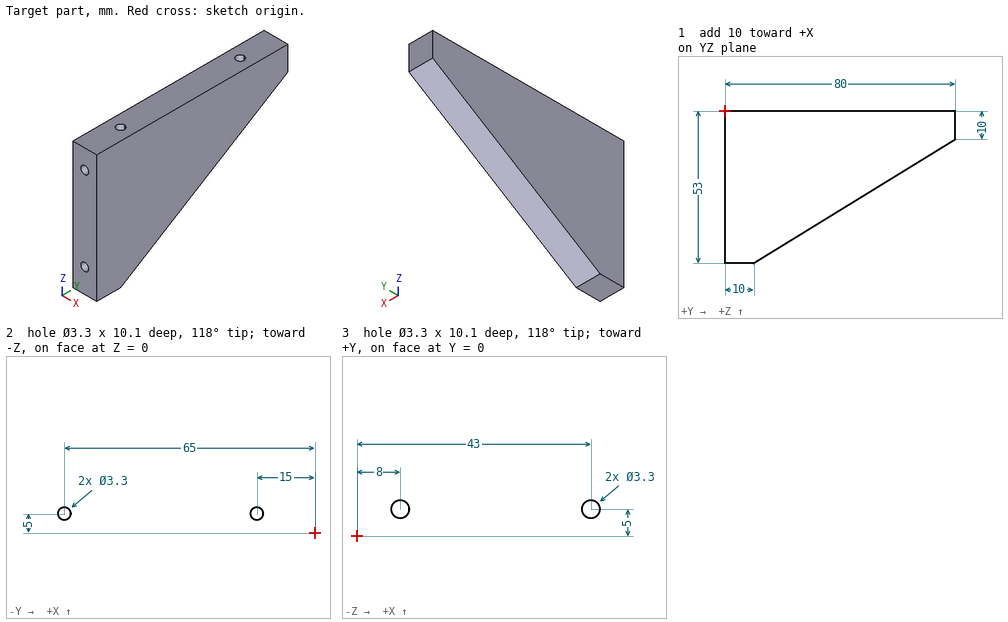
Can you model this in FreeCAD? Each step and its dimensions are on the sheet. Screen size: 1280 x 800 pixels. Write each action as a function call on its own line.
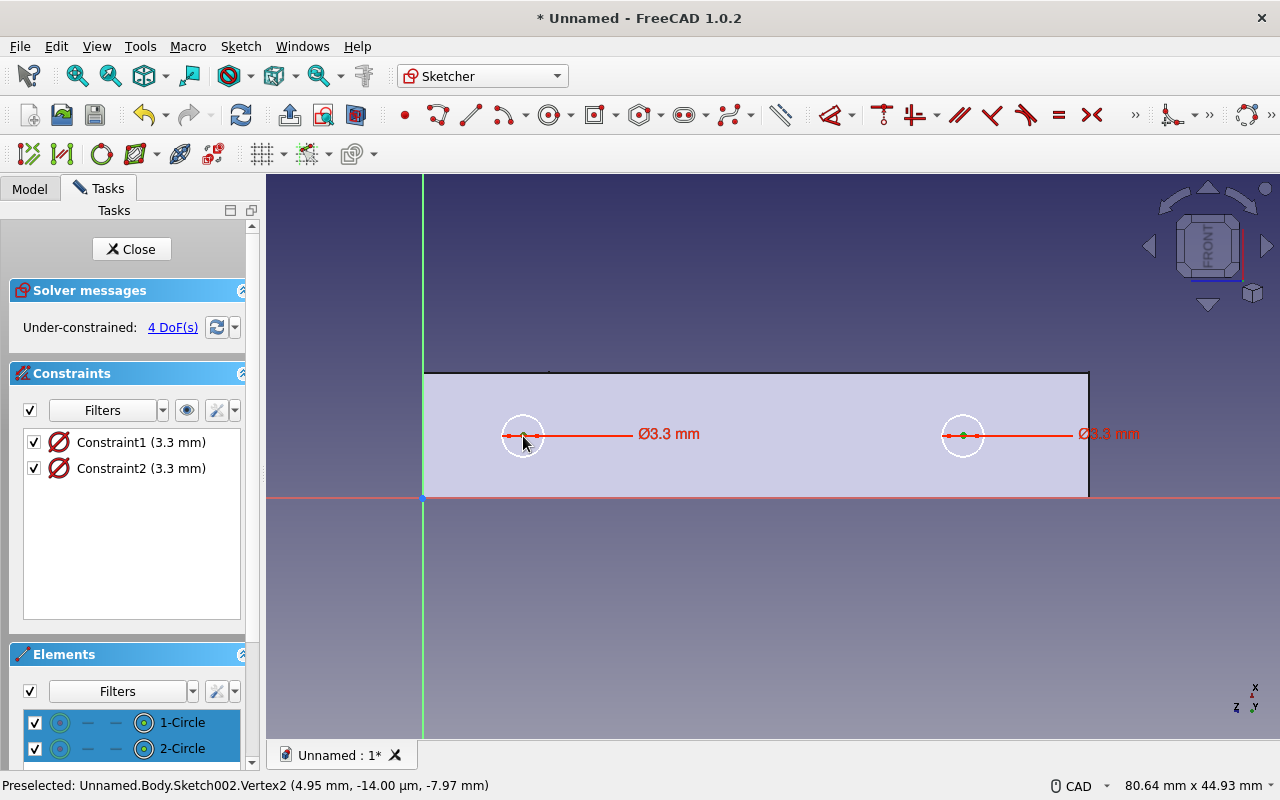
key(h)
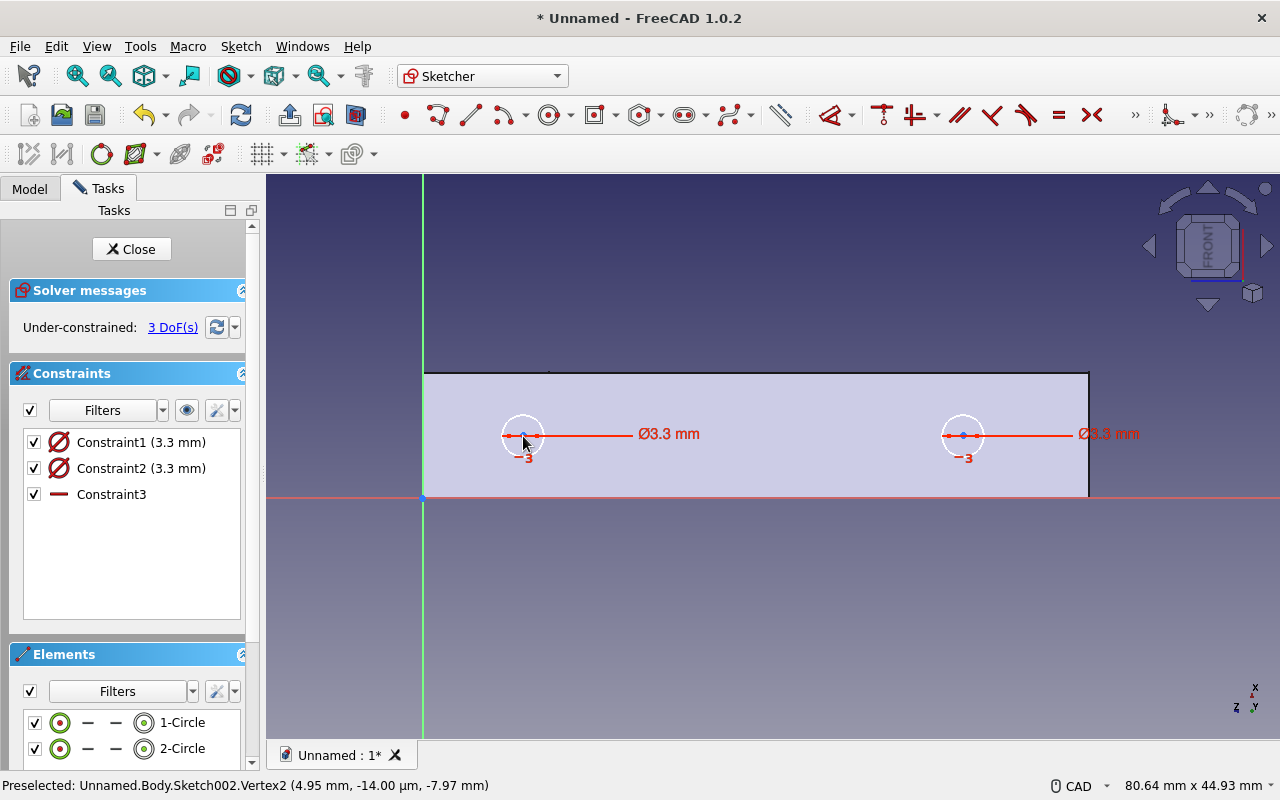
click(830, 116)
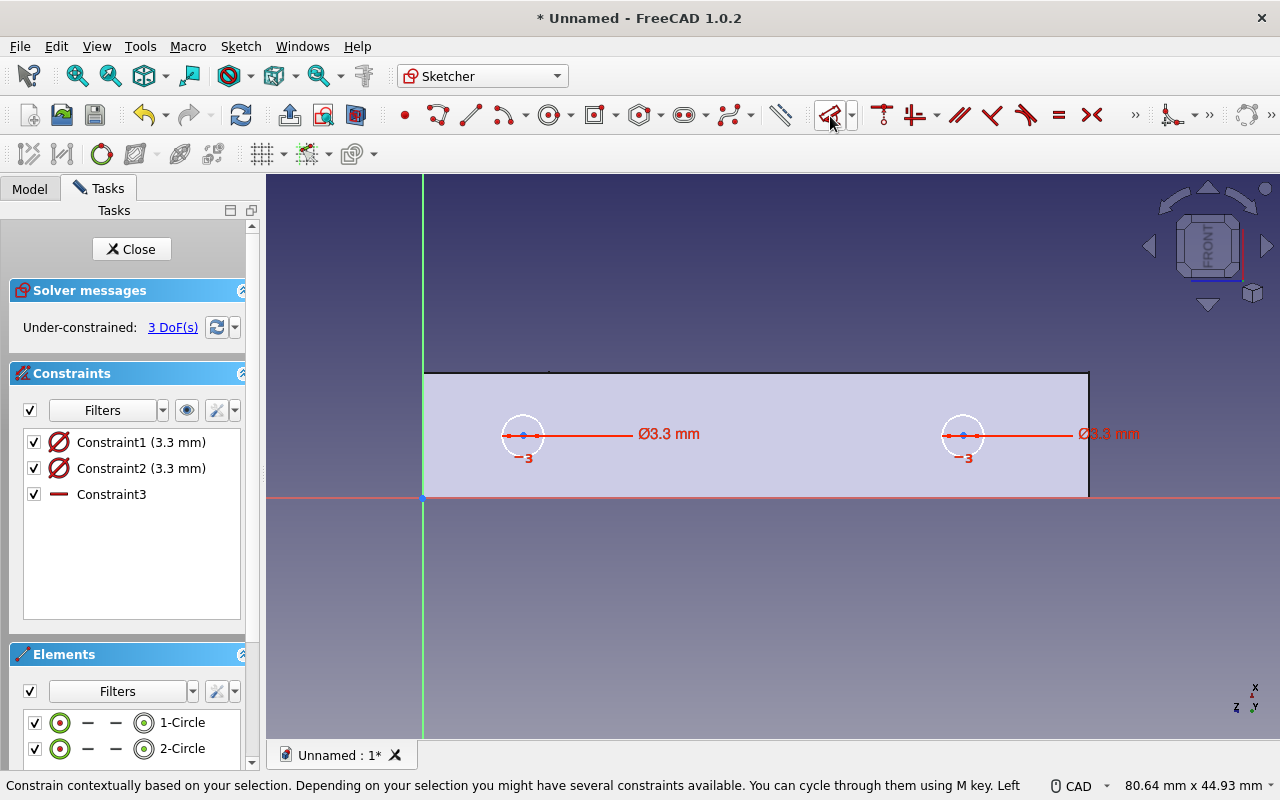
click(963, 436)
click(389, 467)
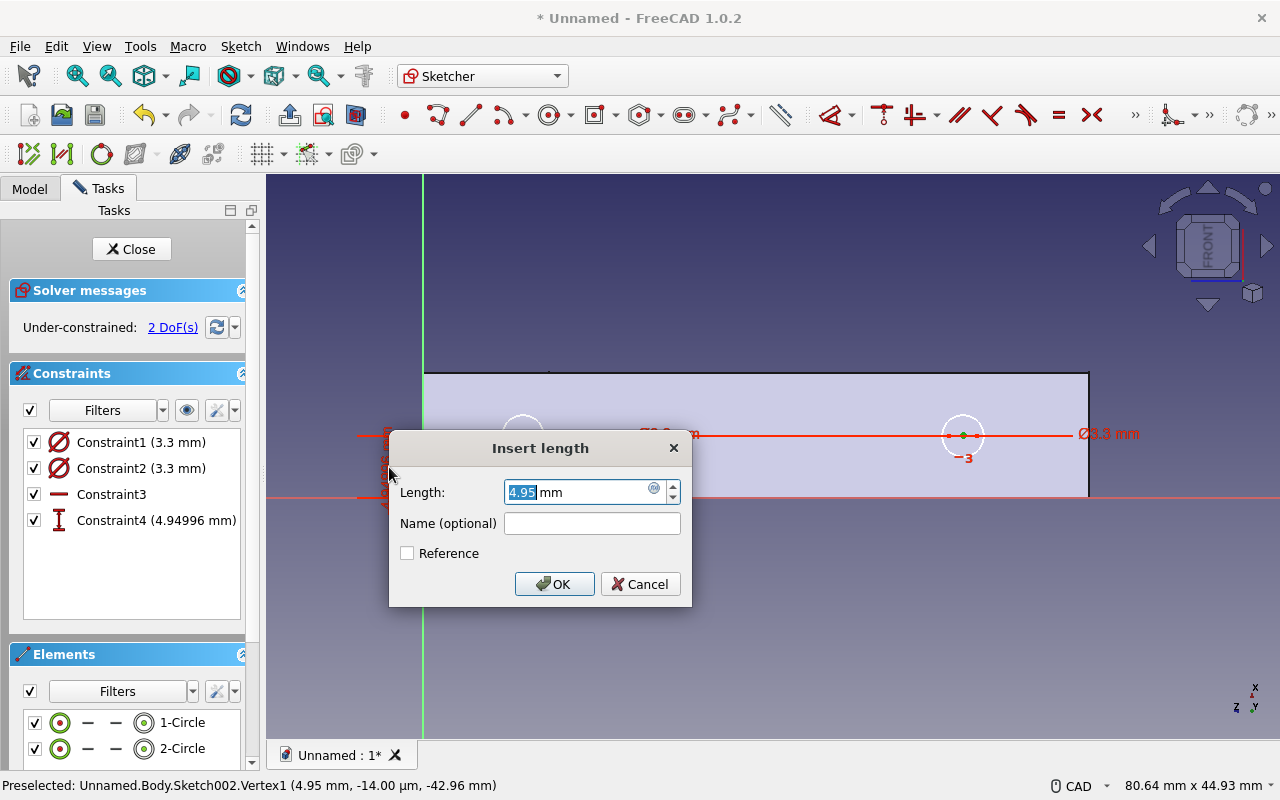
text(5)
key(Return)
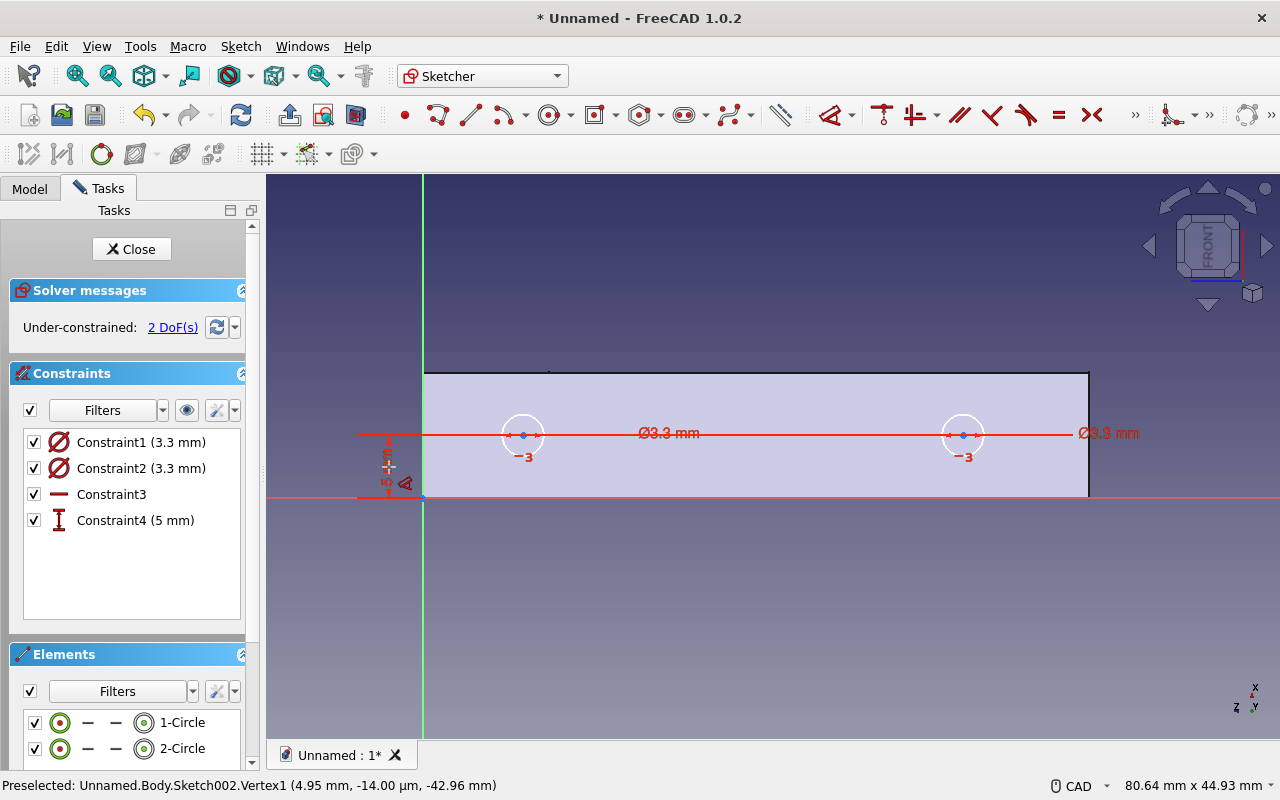
click(523, 435)
click(473, 532)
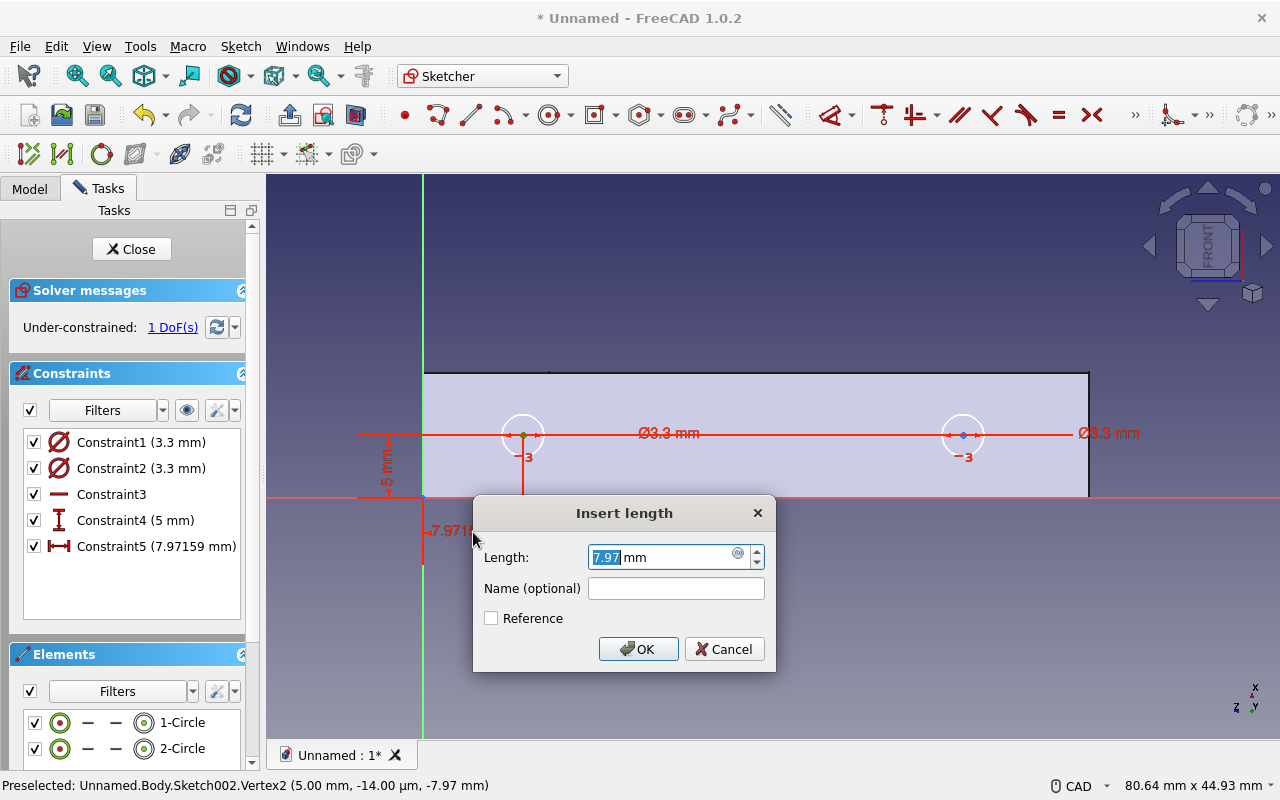
text(8)
key(Return)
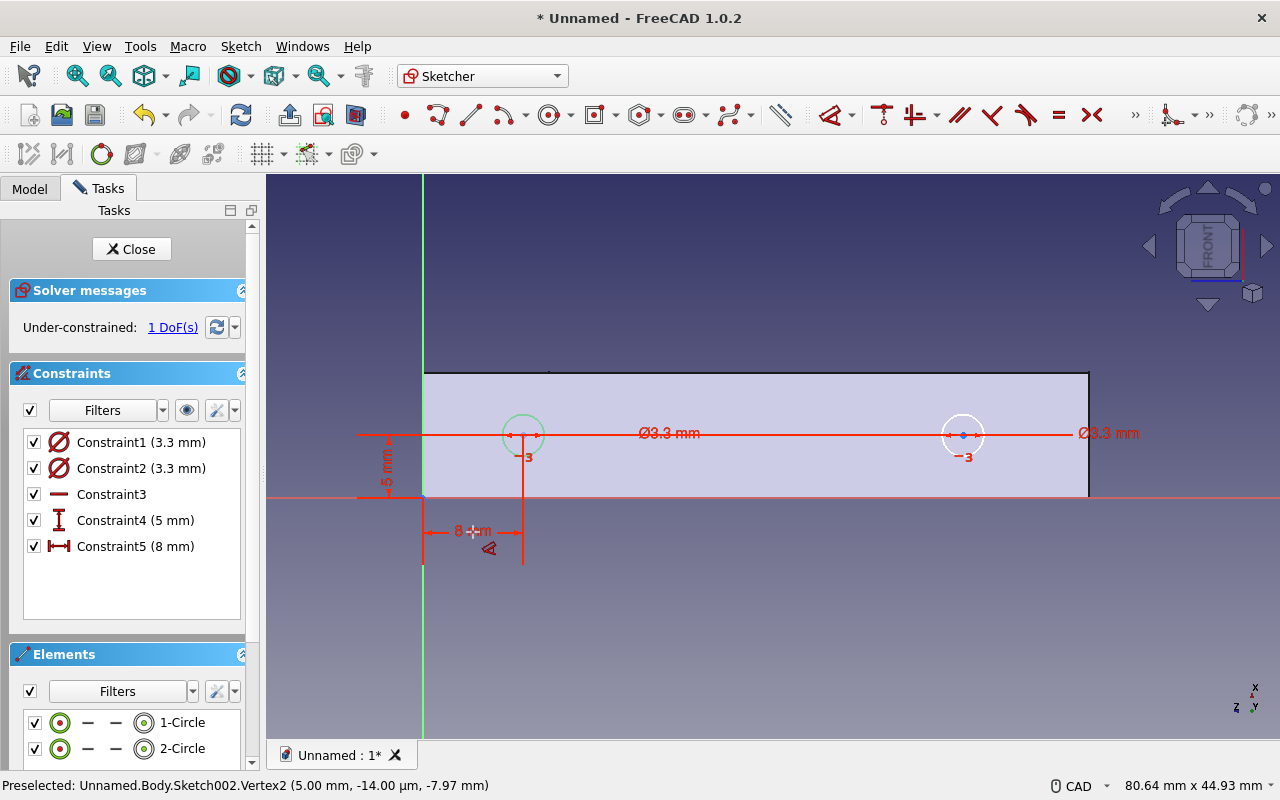
click(963, 435)
click(693, 532)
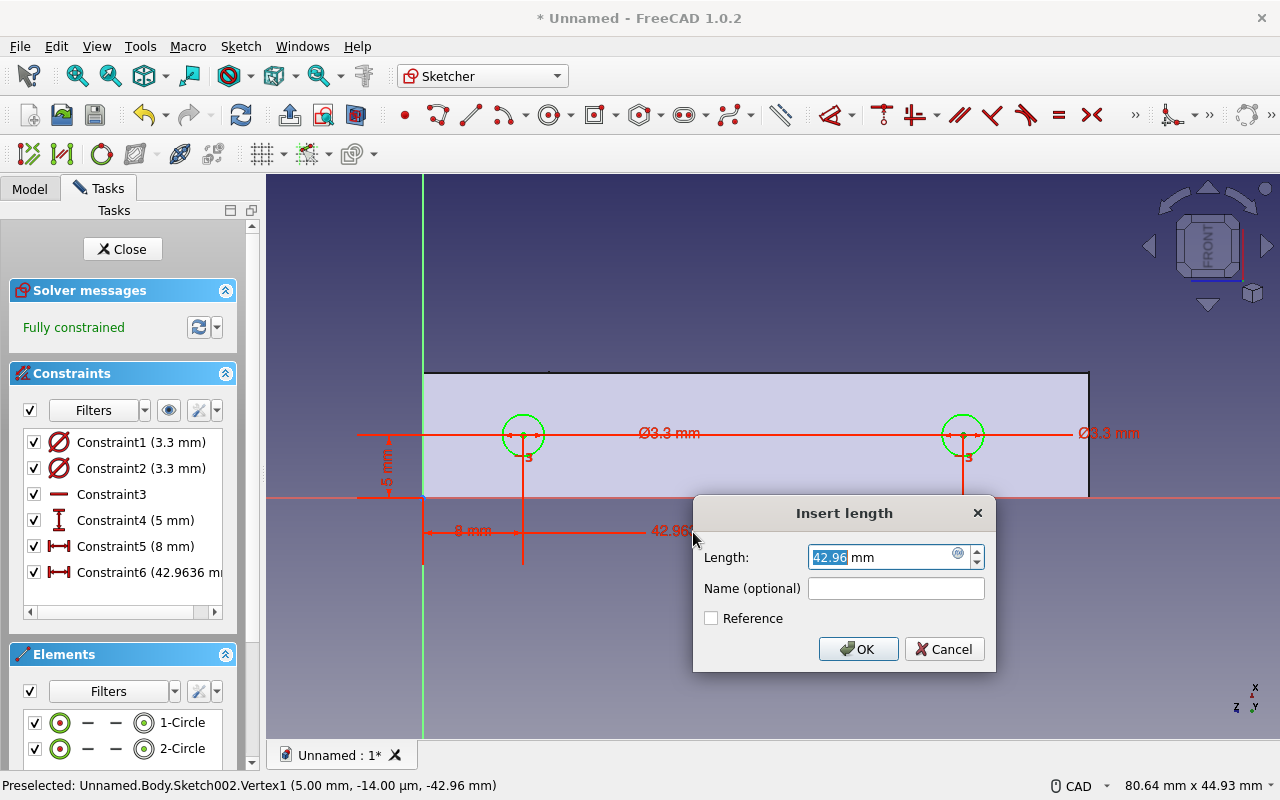
text(43)
key(Return)
key(Escape)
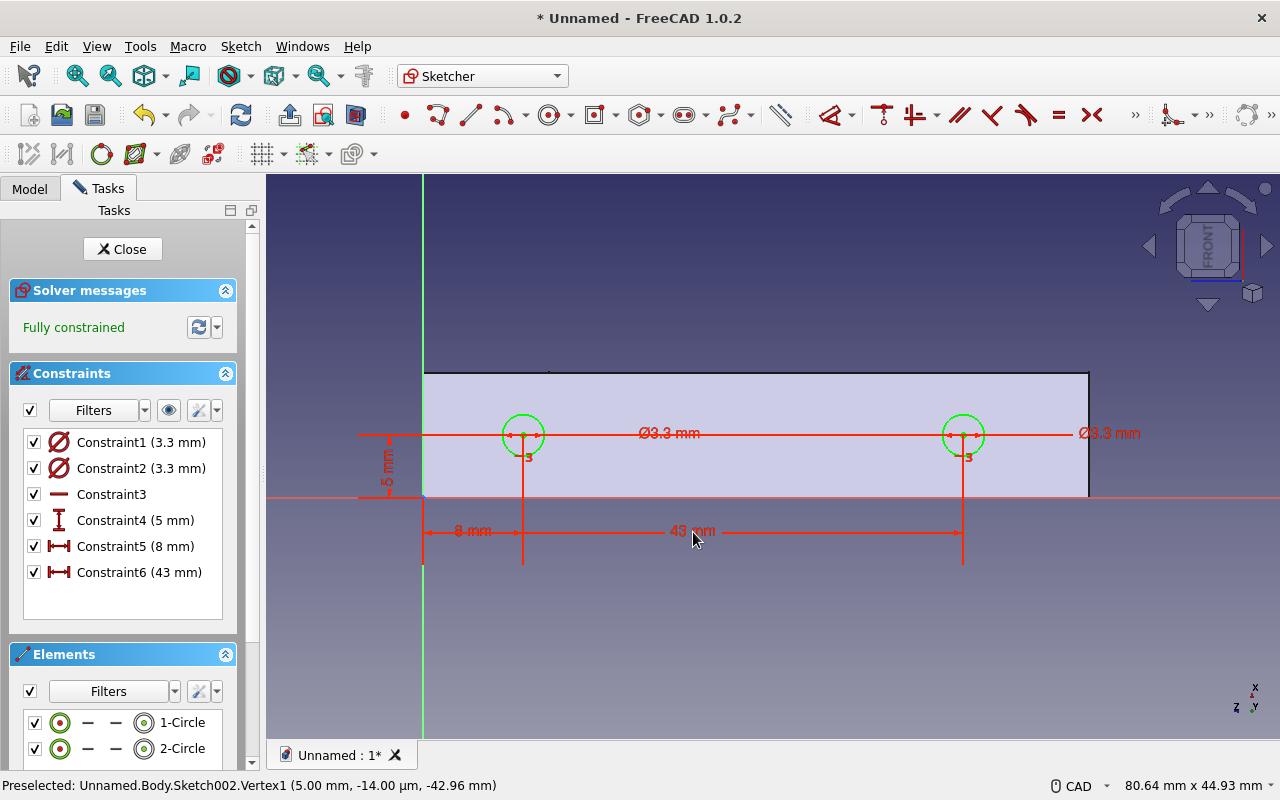
click(123, 249)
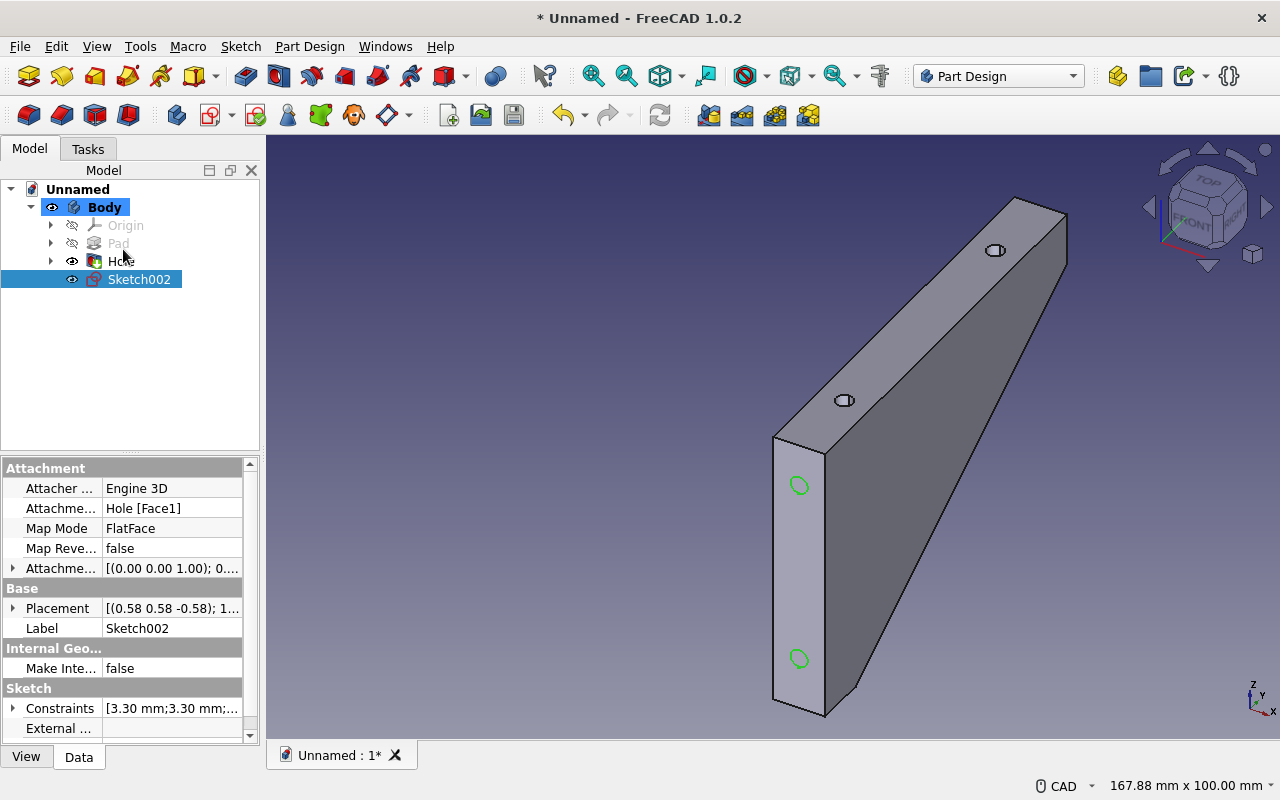
click(279, 76)